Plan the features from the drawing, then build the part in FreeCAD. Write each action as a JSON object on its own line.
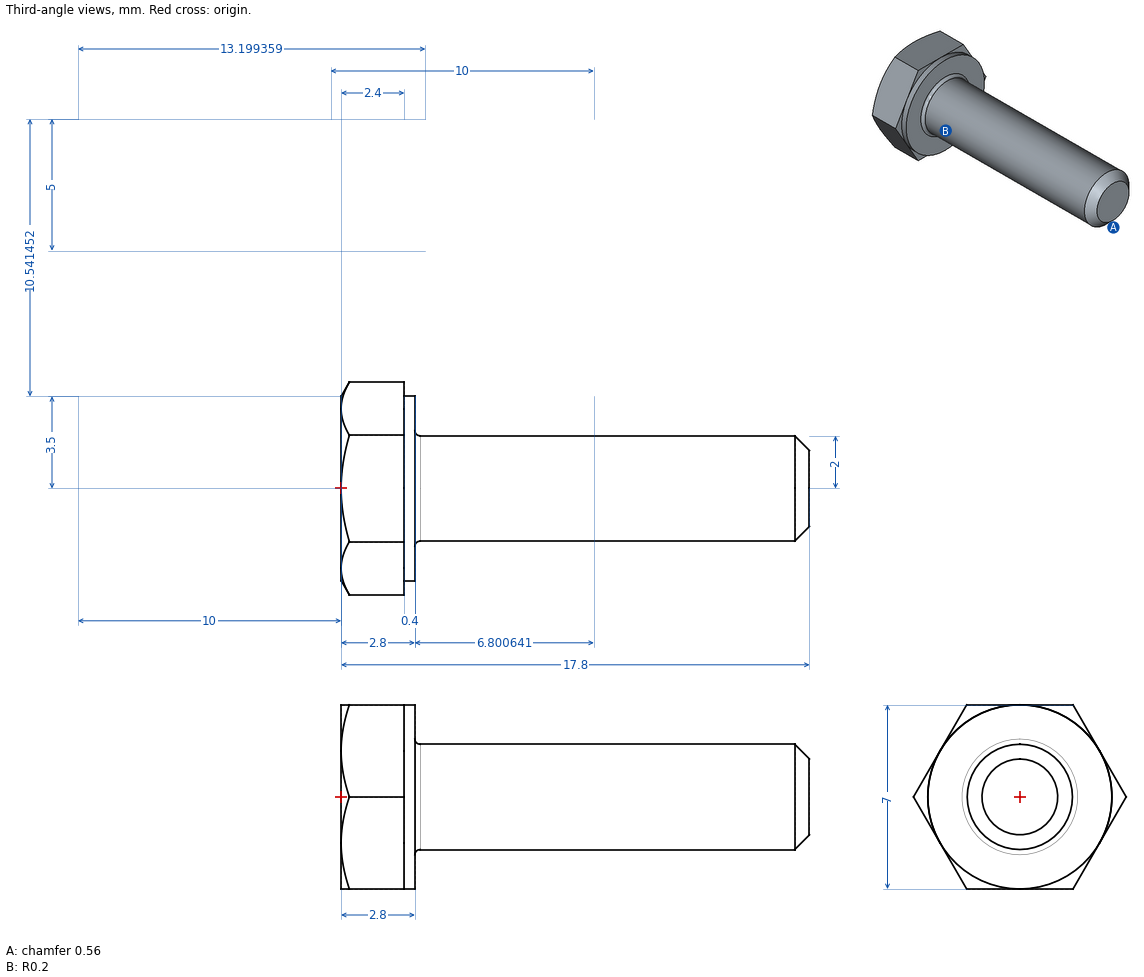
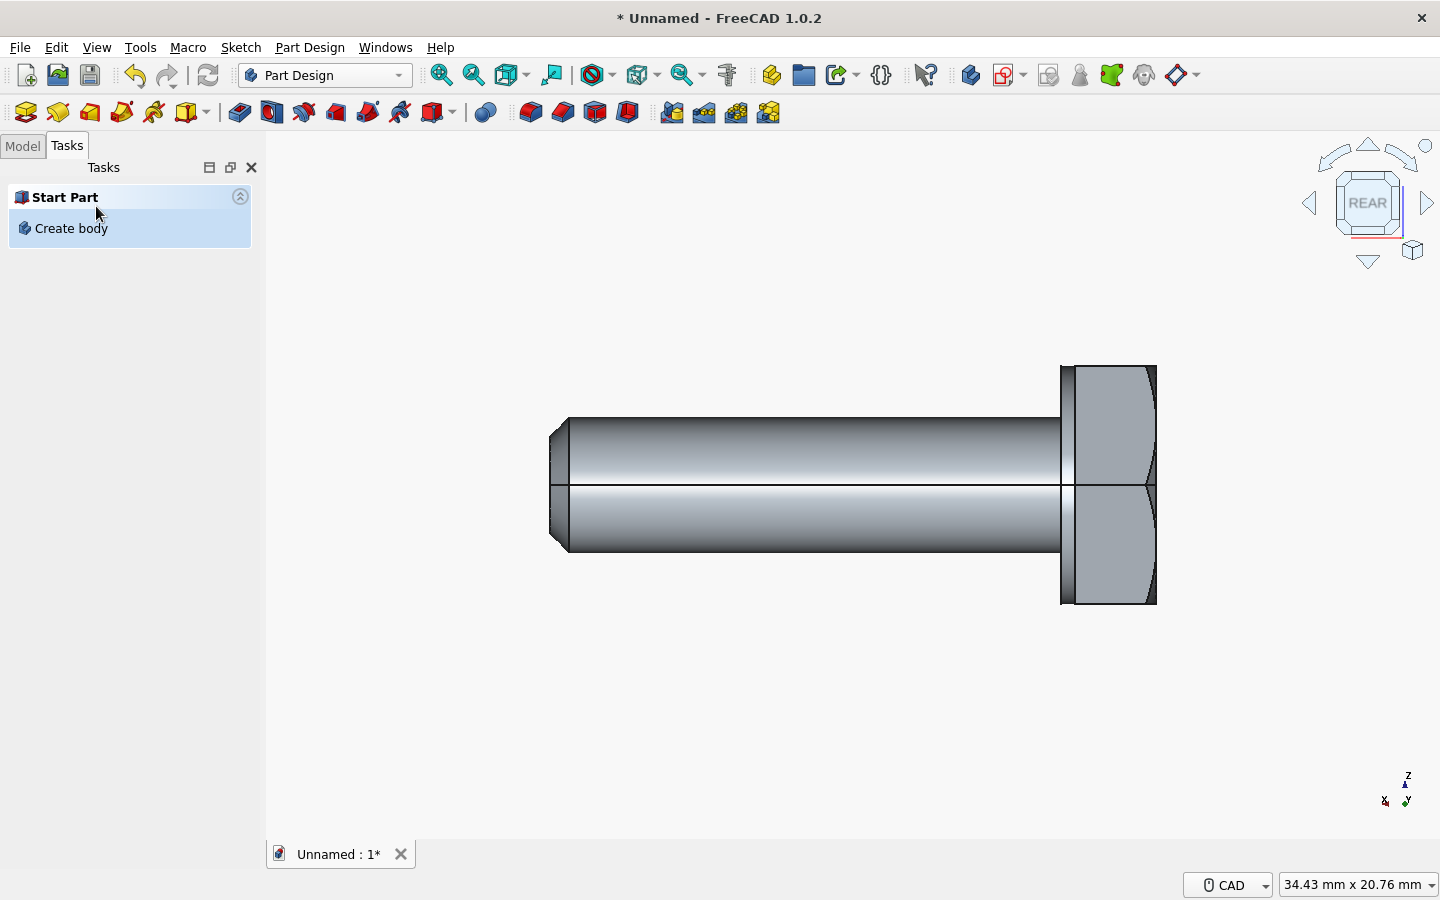
{"action": "key", "text": "6"}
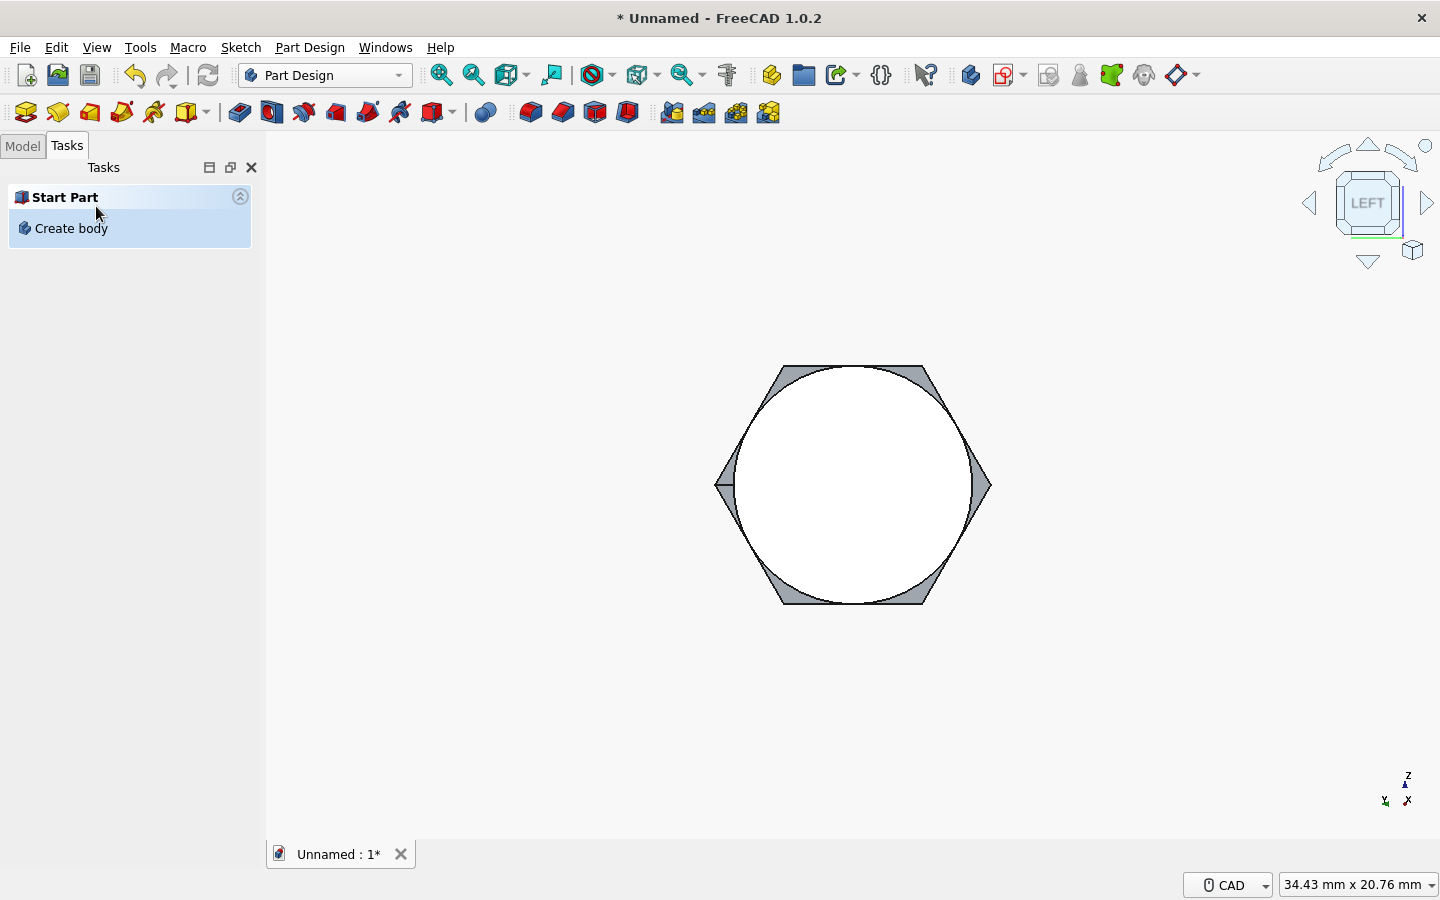
{"action": "left_click", "coordinate": [442, 76]}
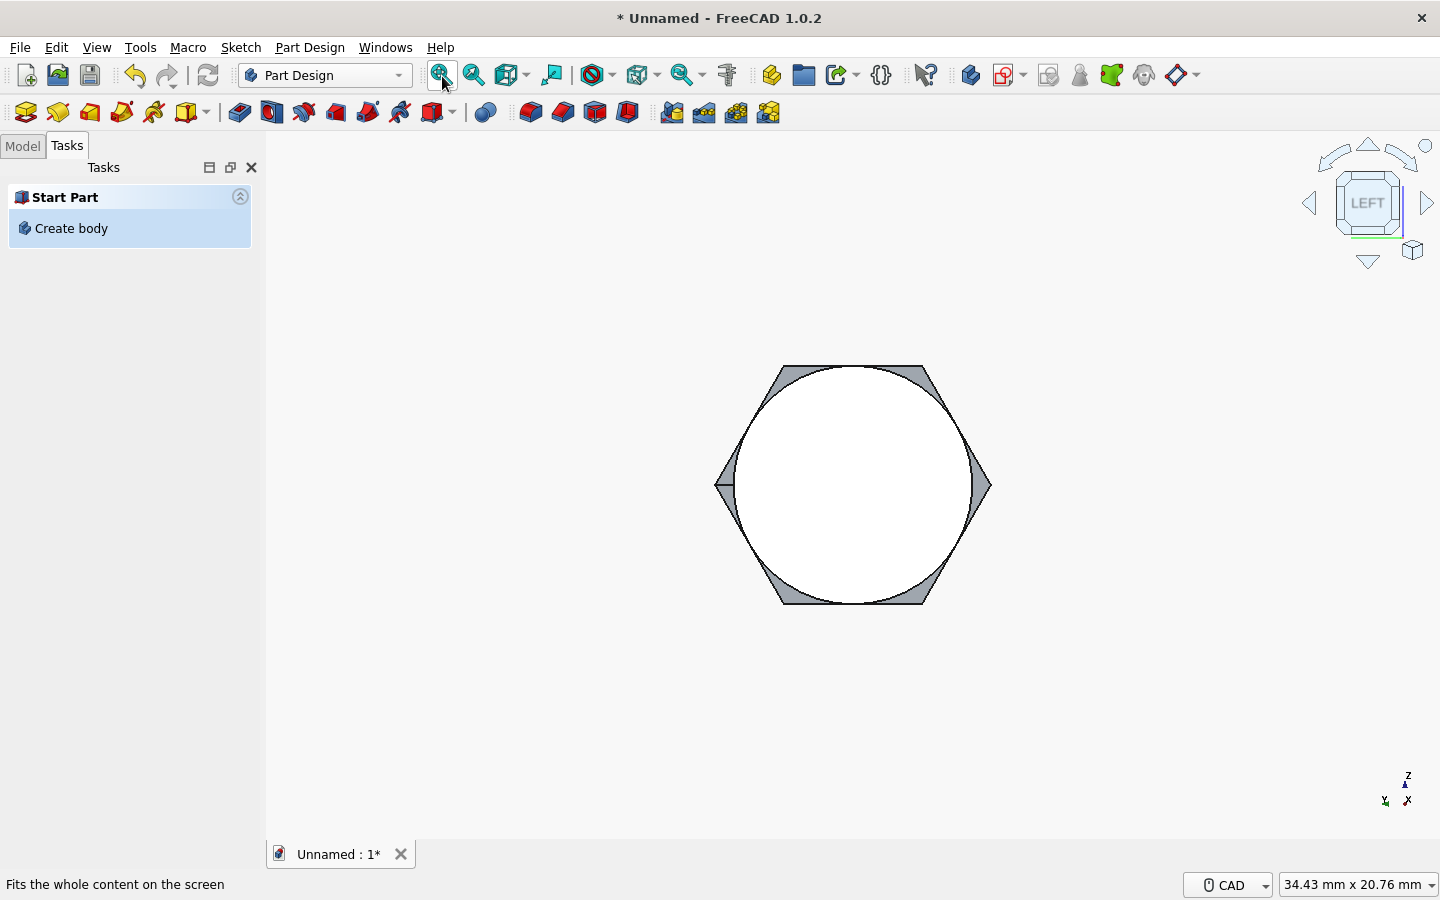
{"action": "key", "text": "v 3"}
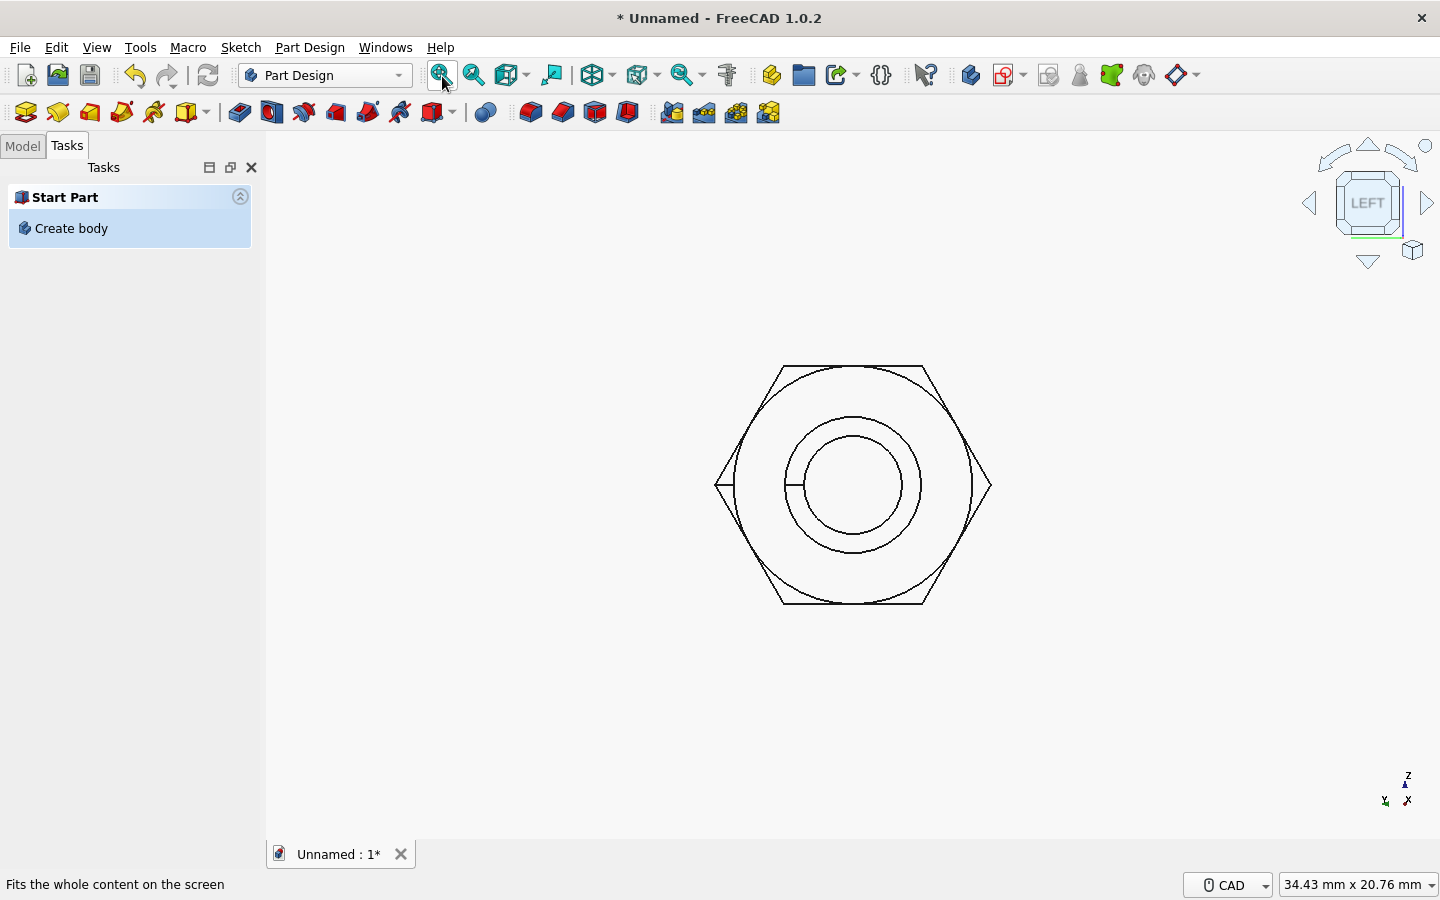
{"action": "key", "text": "0"}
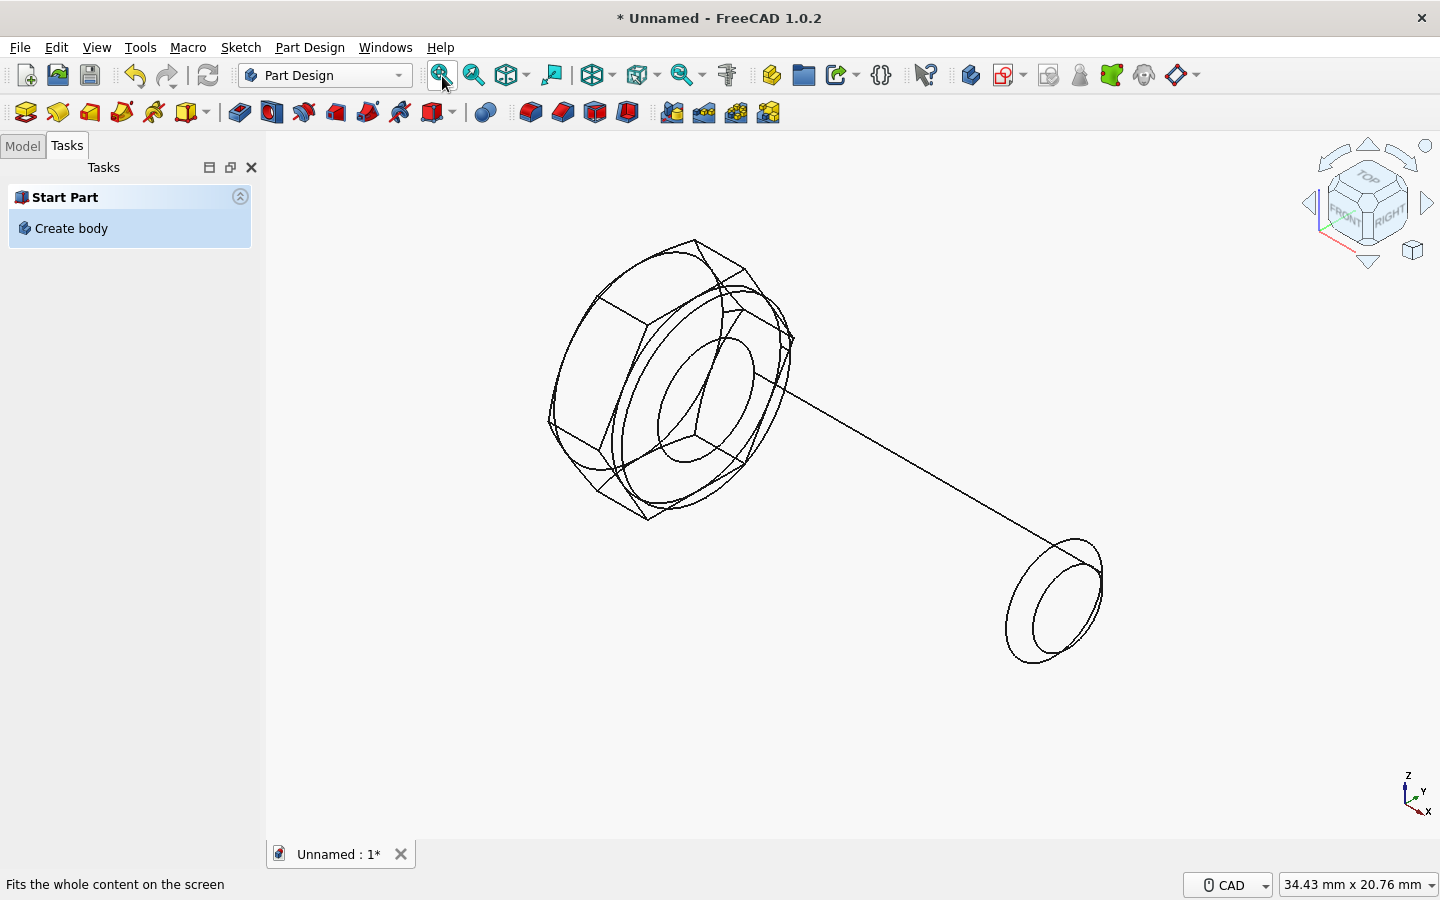
{"action": "left_click", "coordinate": [658, 427]}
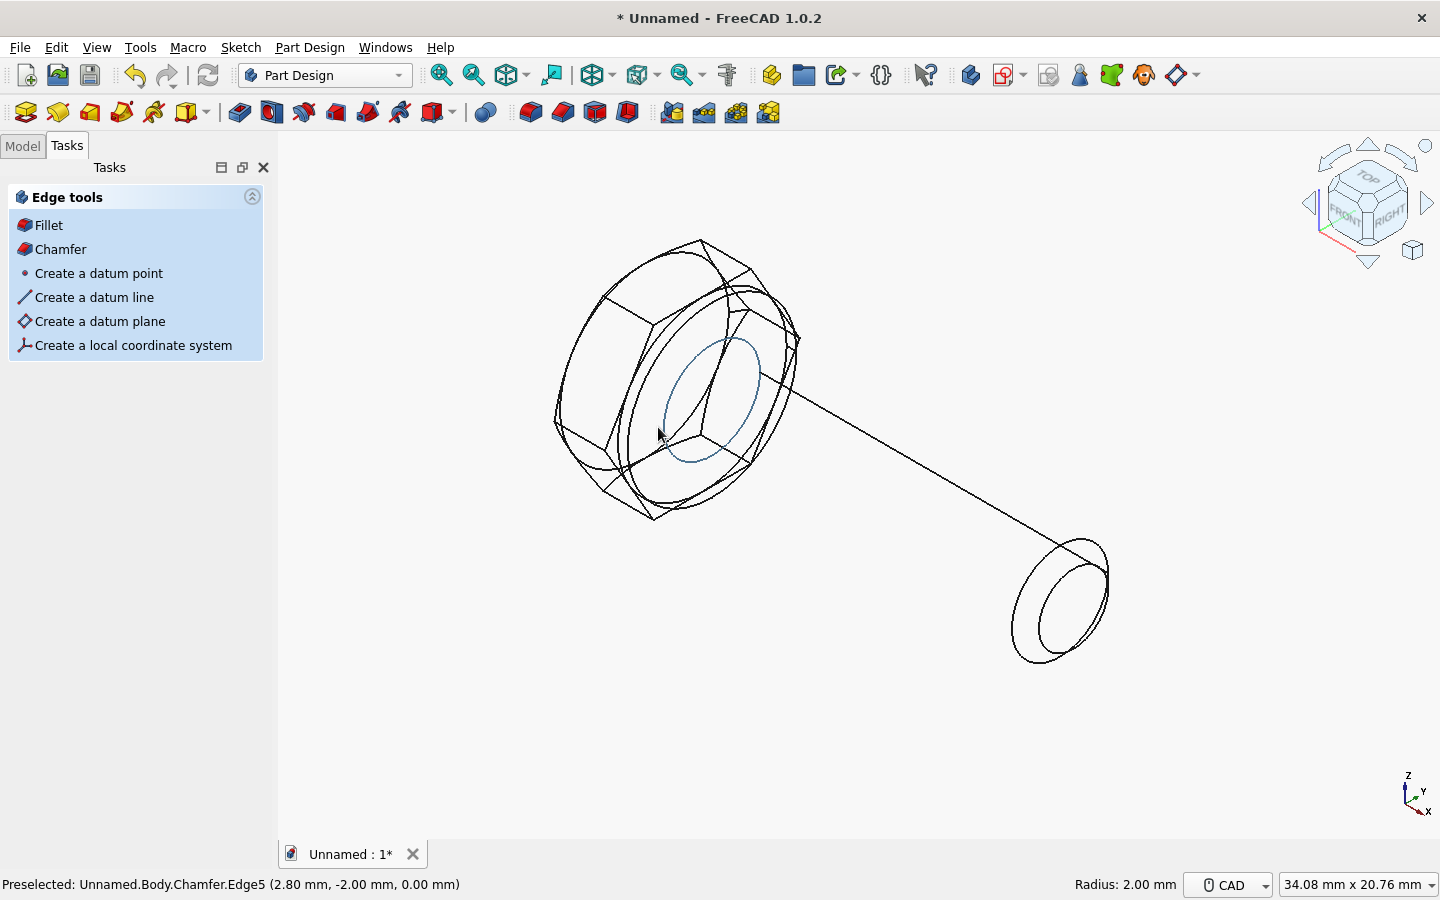
{"action": "key", "text": "v 1"}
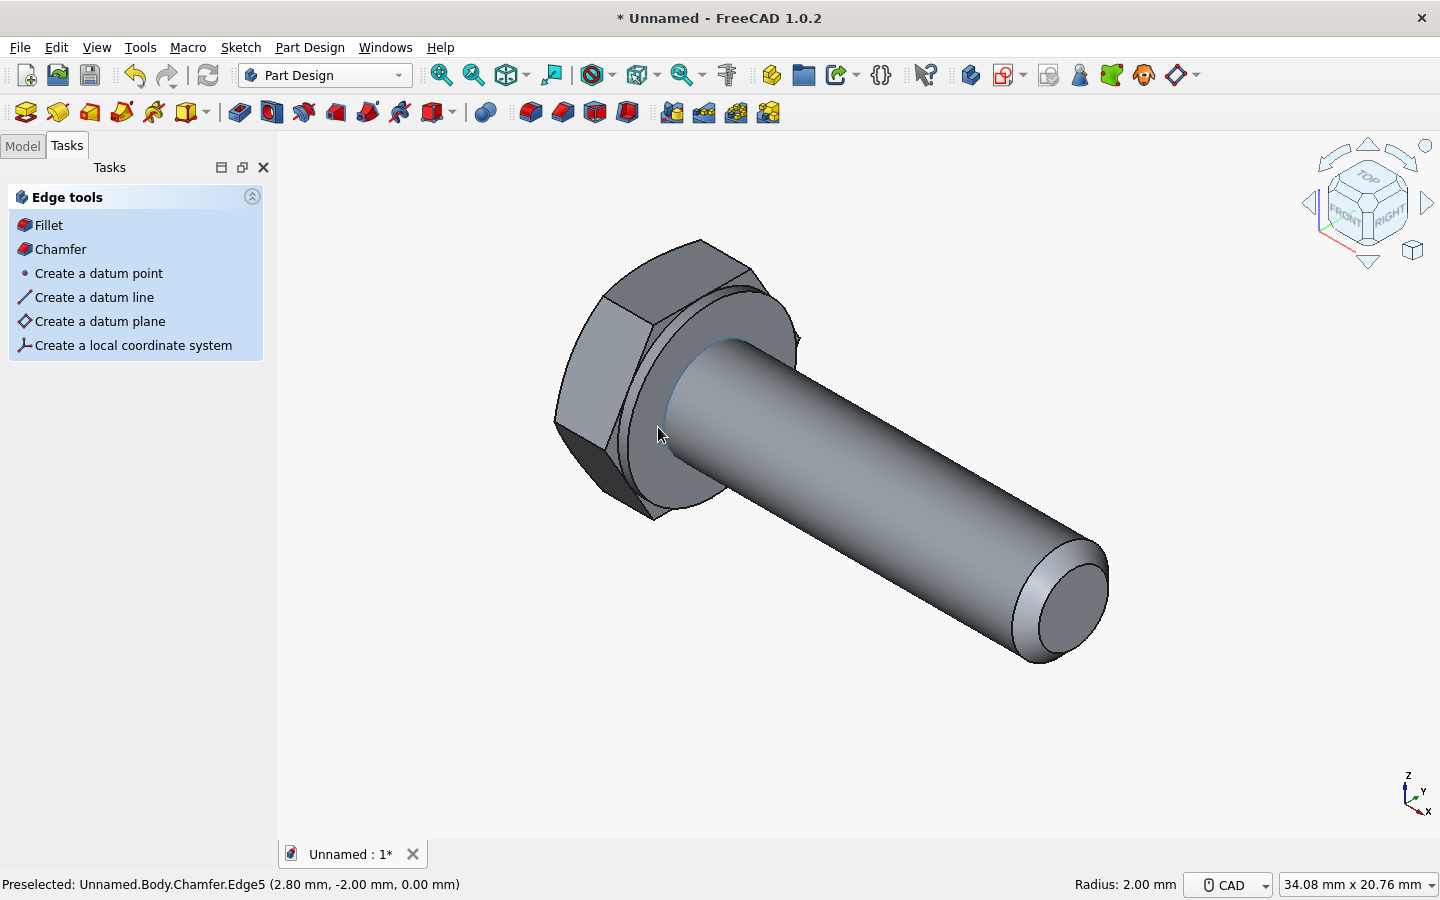
{"action": "left_click", "coordinate": [532, 112]}